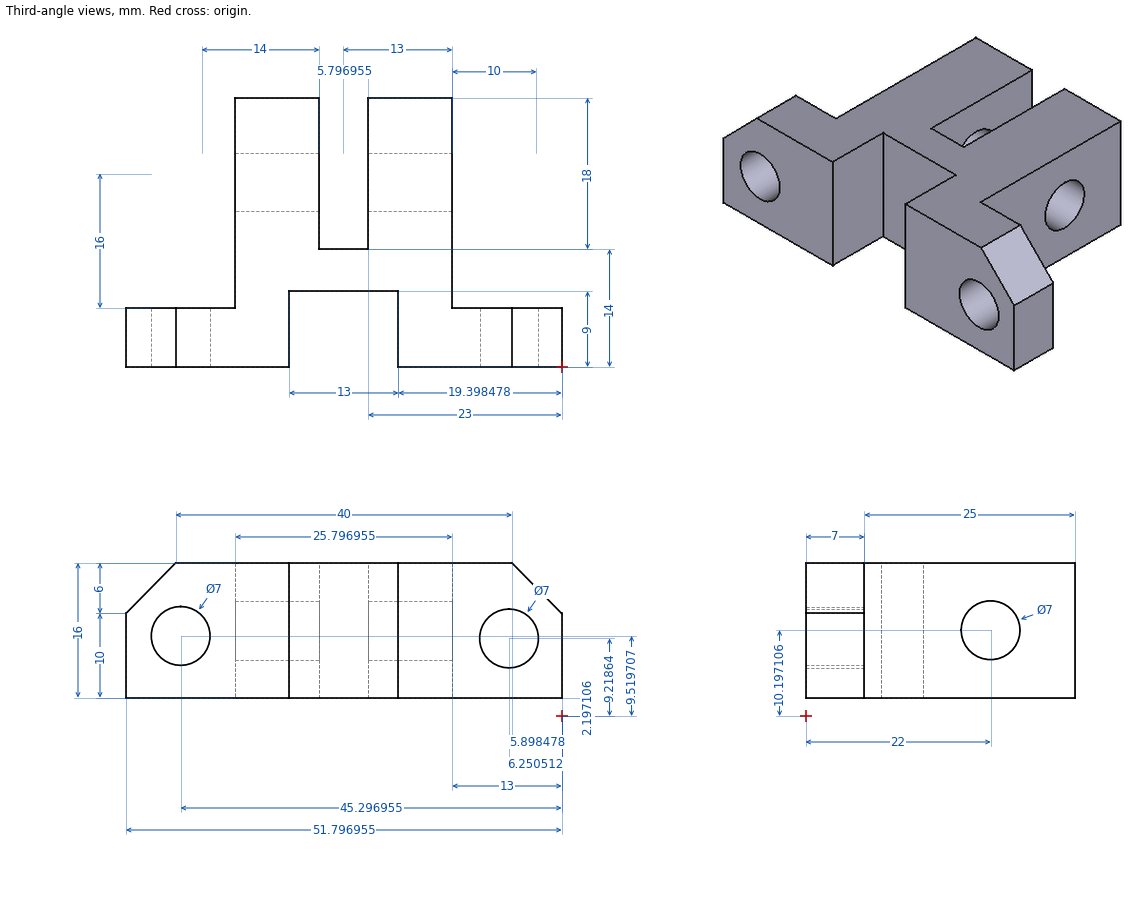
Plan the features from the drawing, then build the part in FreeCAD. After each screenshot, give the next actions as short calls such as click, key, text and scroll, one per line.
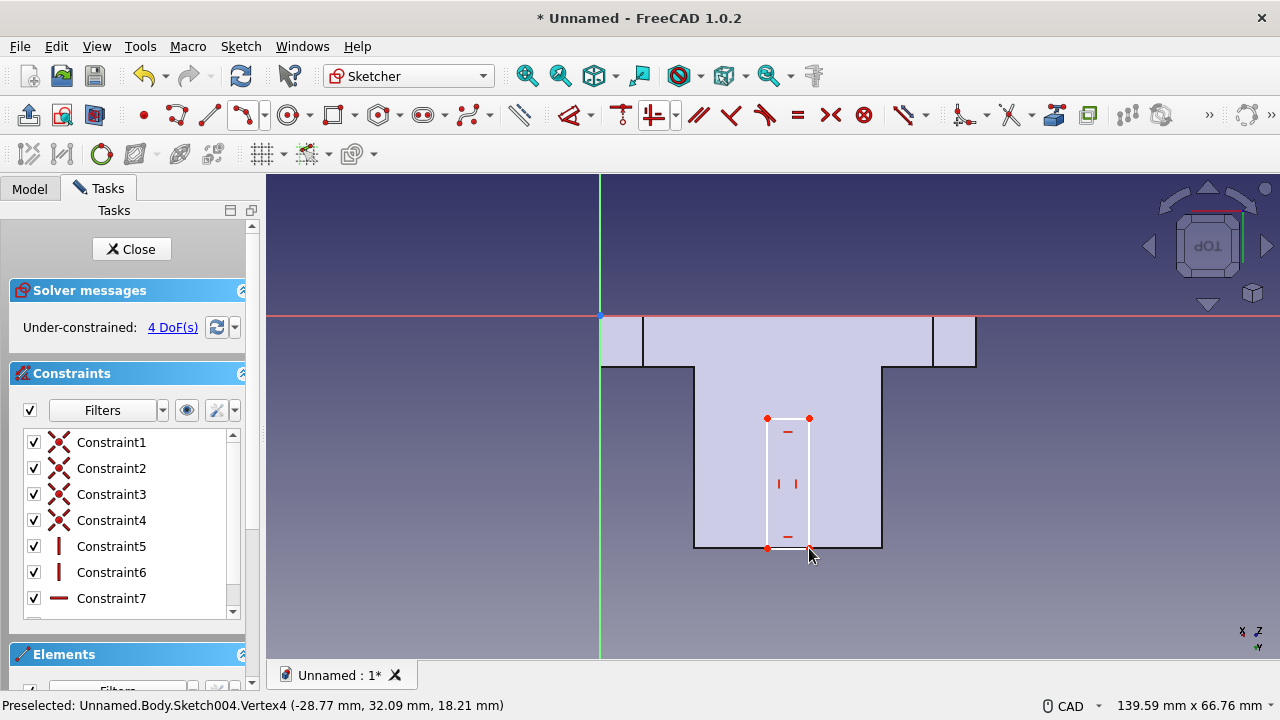
key(d)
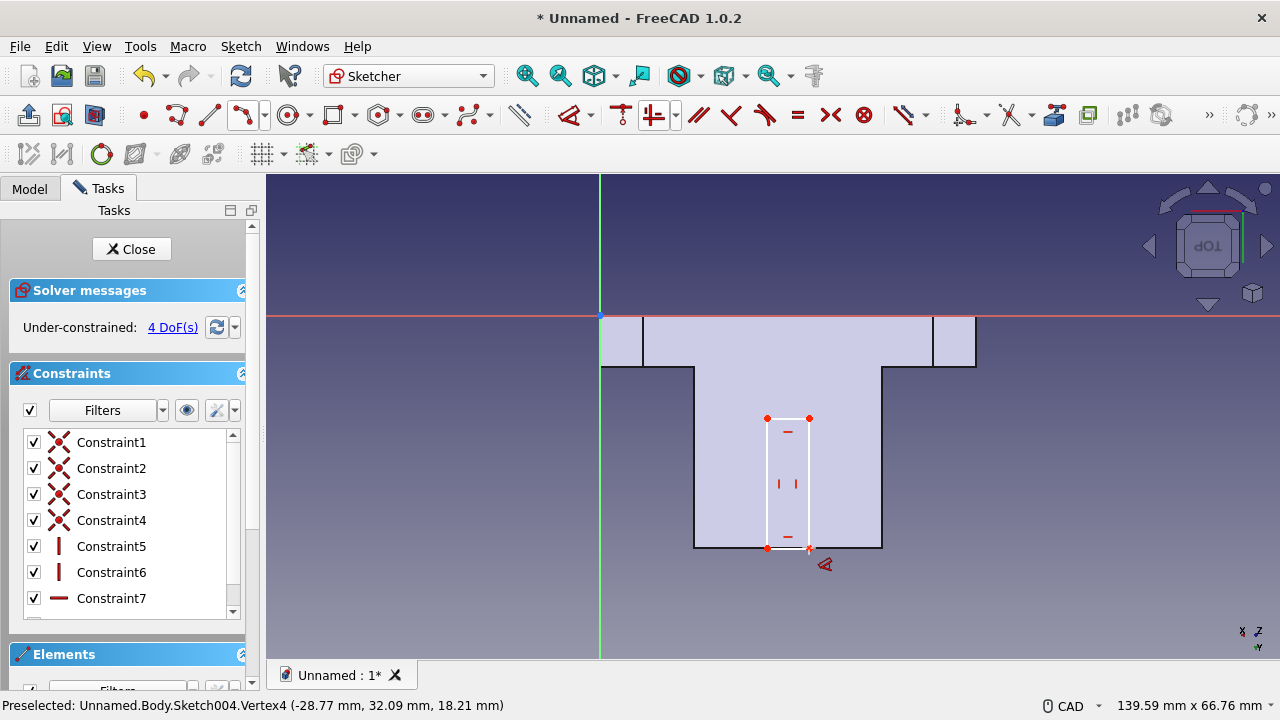
click(767, 458)
click(733, 484)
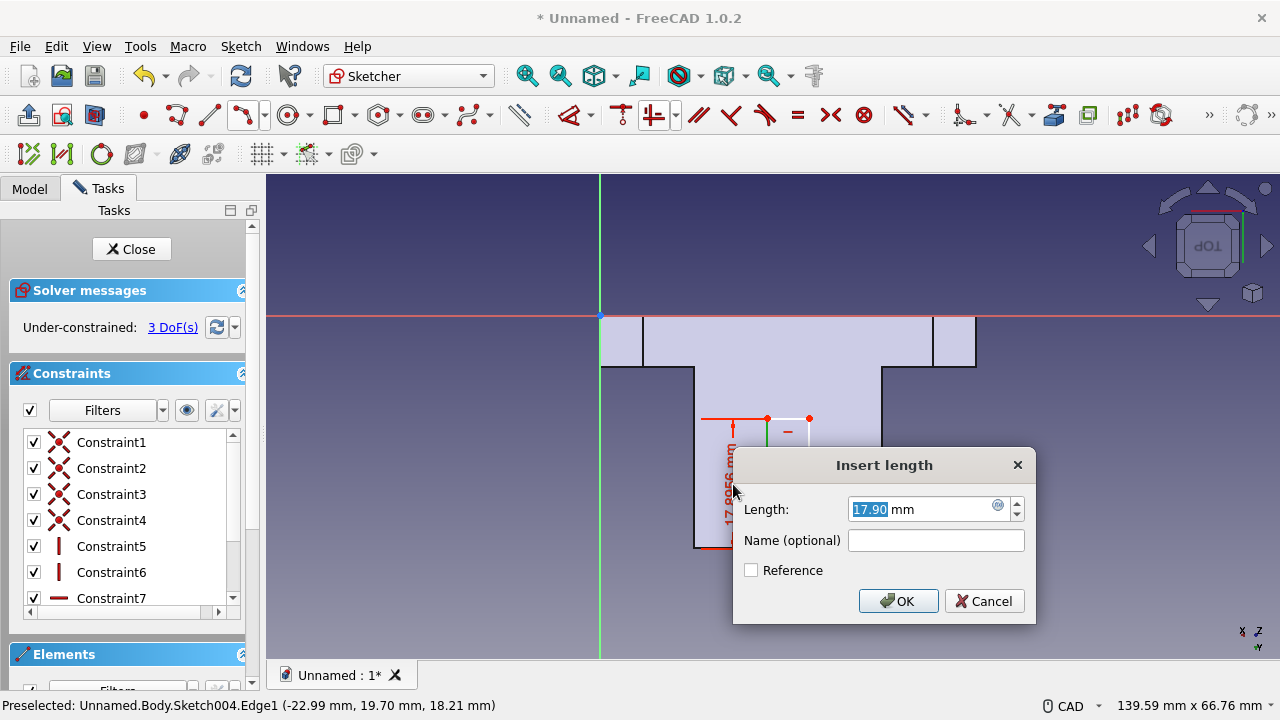
text(18)
key(Return)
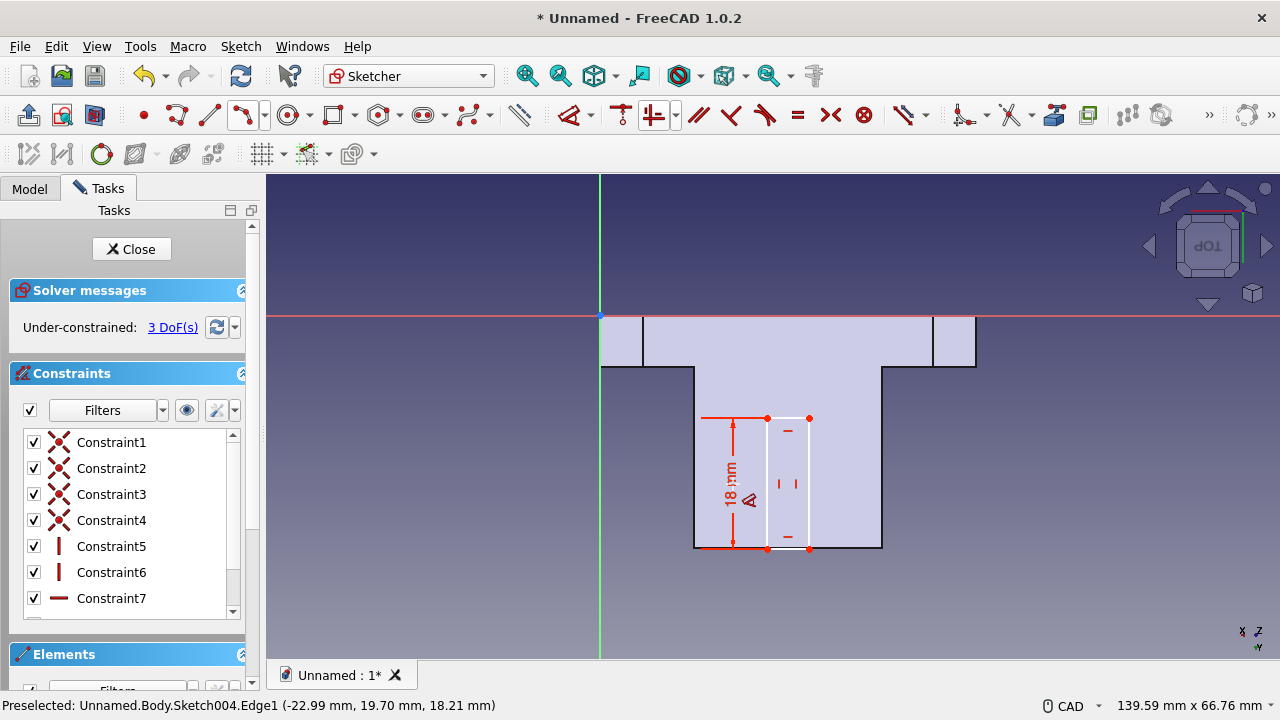
click(767, 418)
click(684, 282)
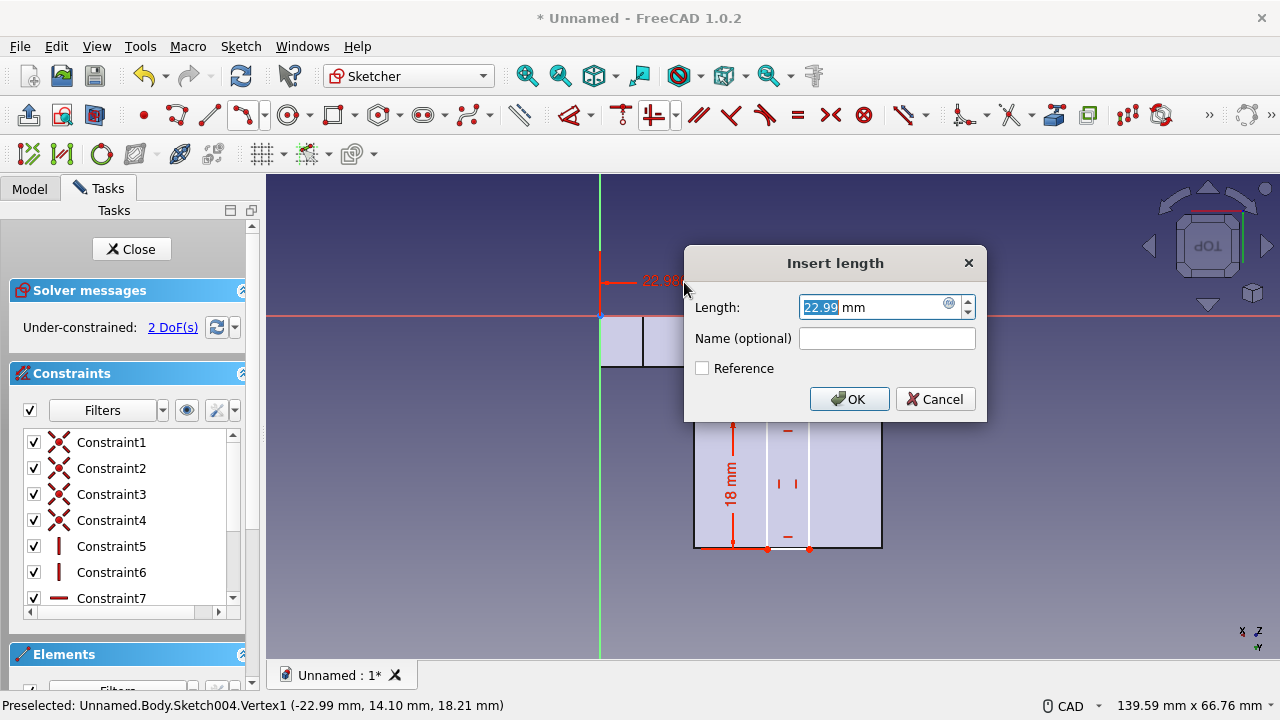
text(23)
key(Return)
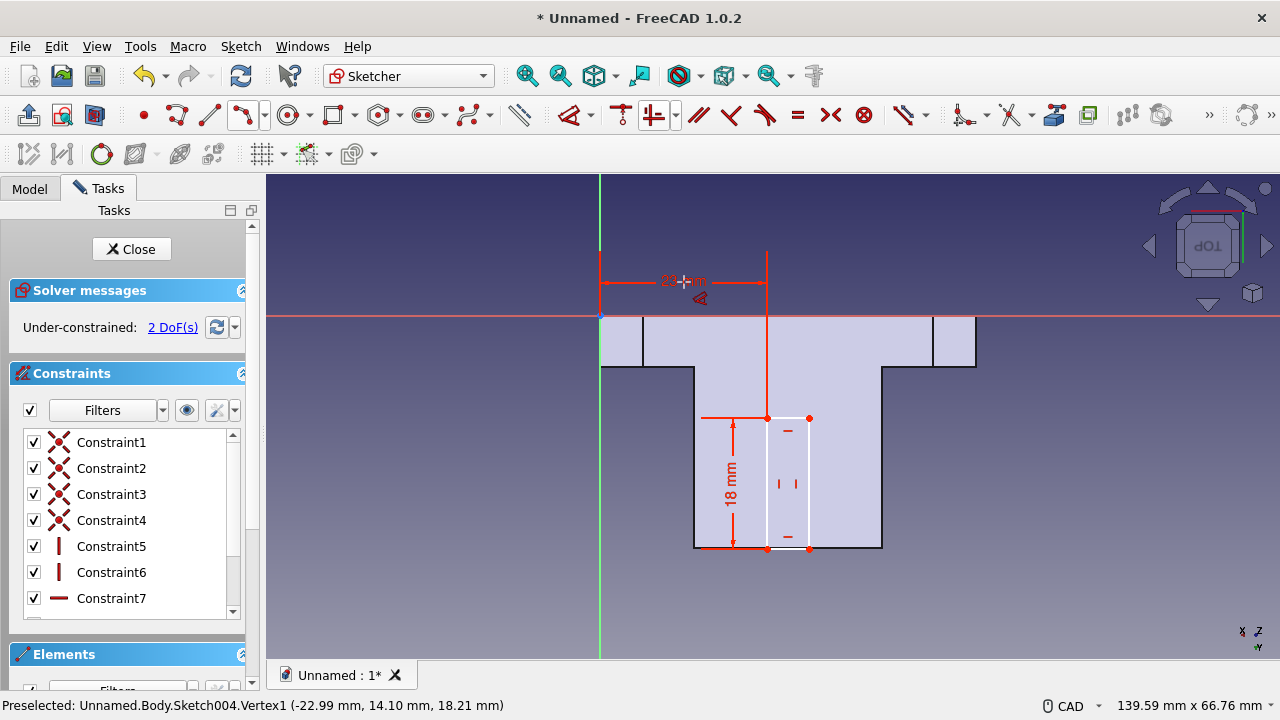
click(767, 418)
click(566, 367)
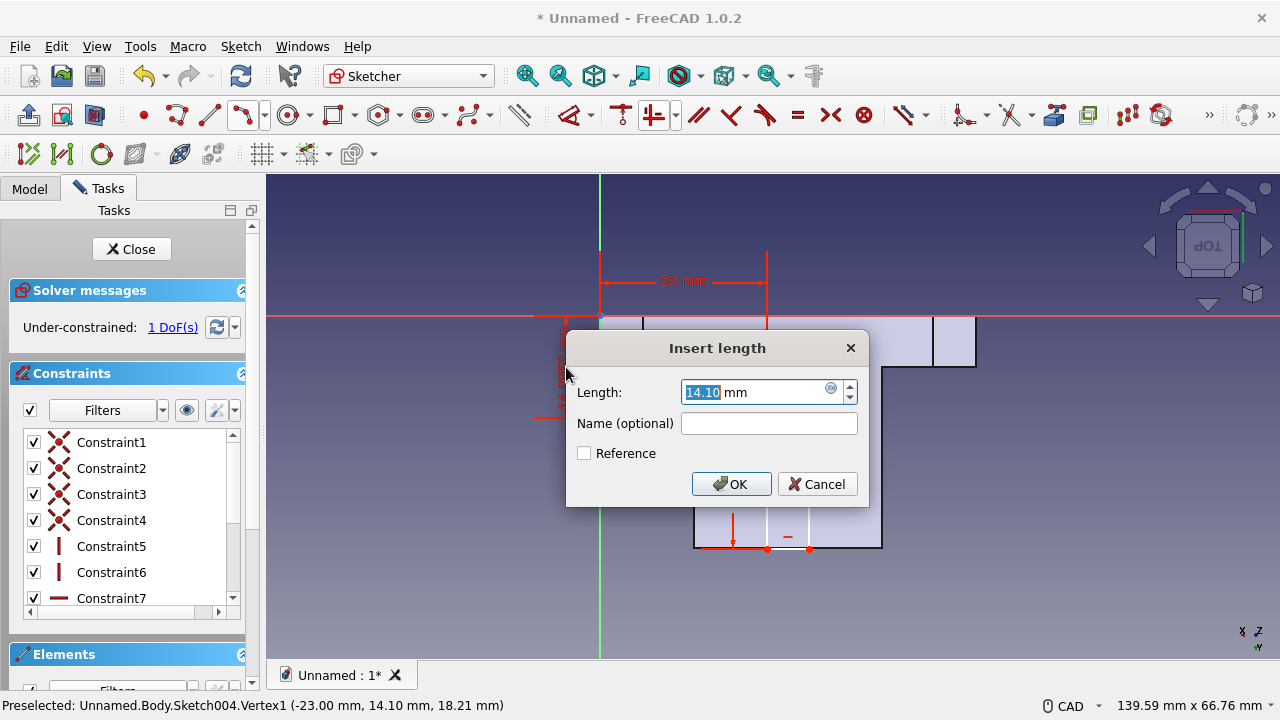
text(14)
key(Return)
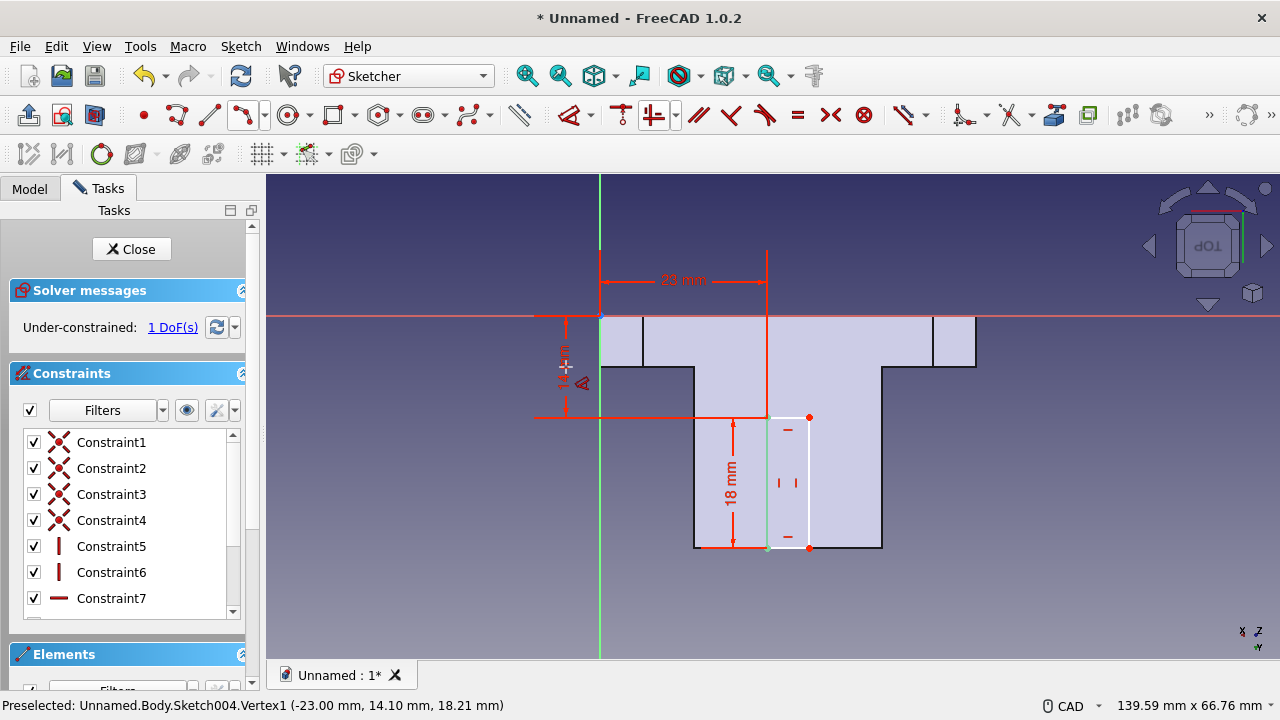
click(780, 548)
click(788, 582)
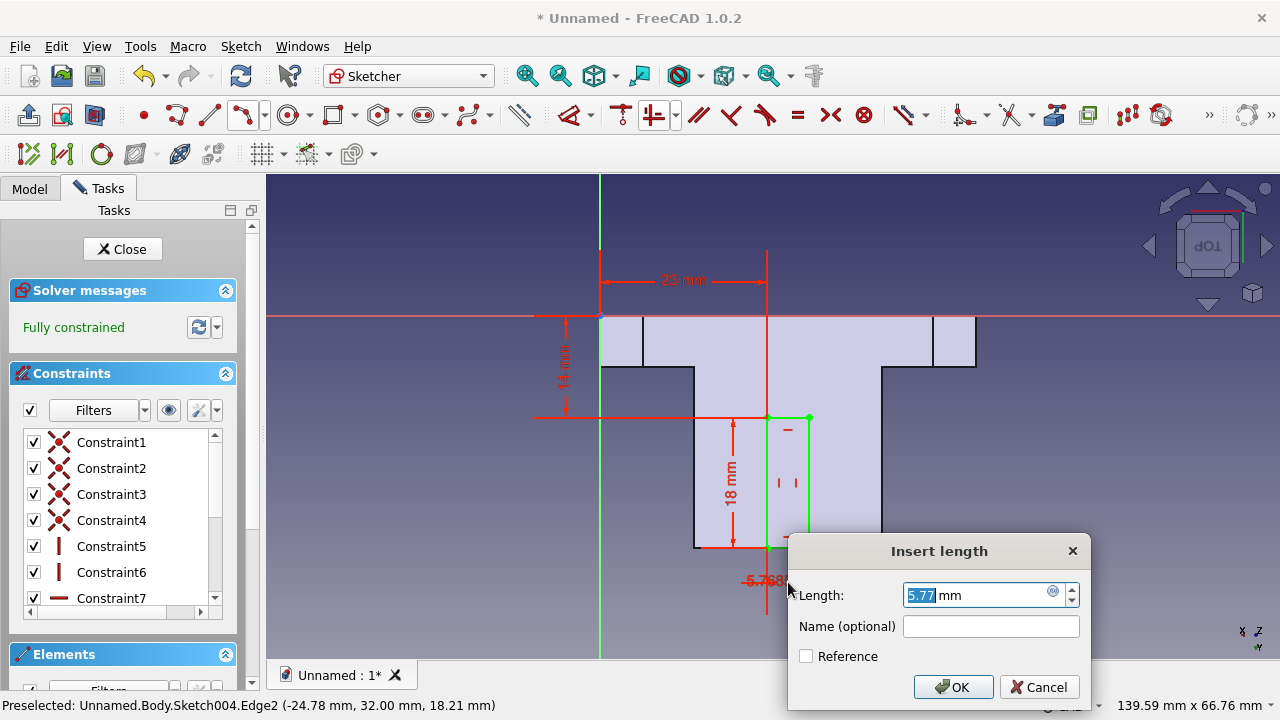
text(5.796955)
key(Return)
key(Escape)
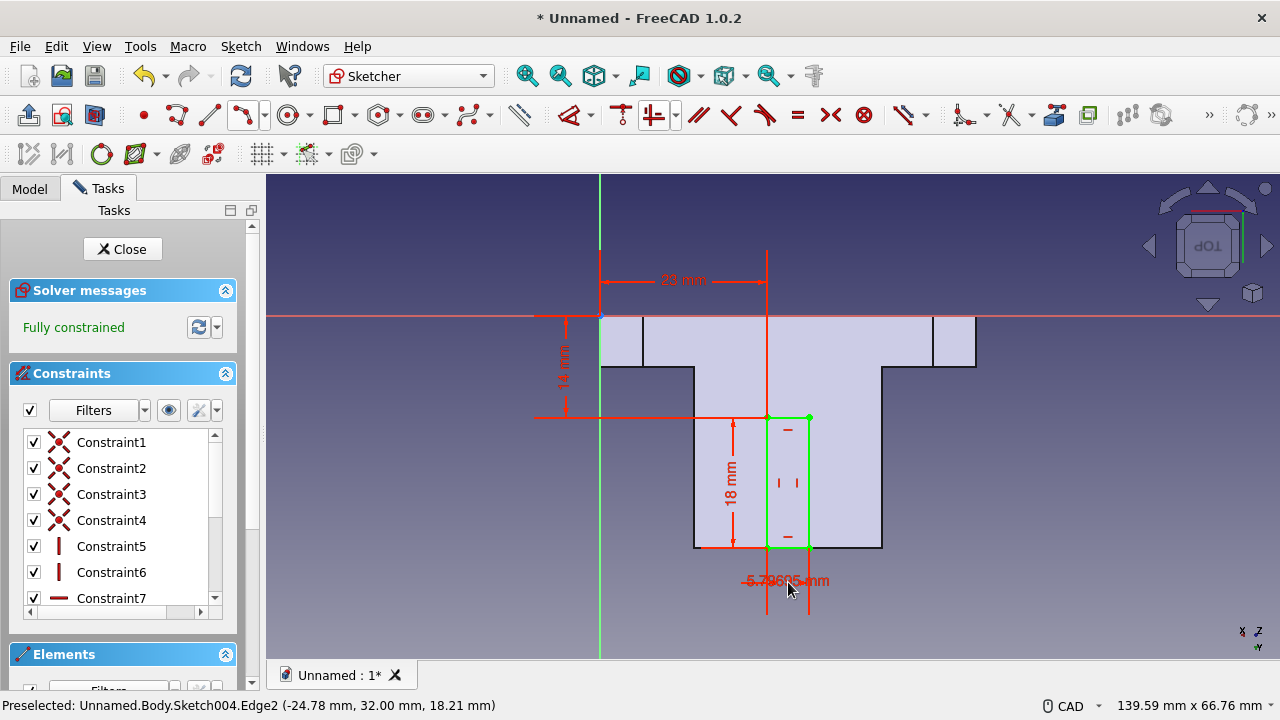
click(123, 249)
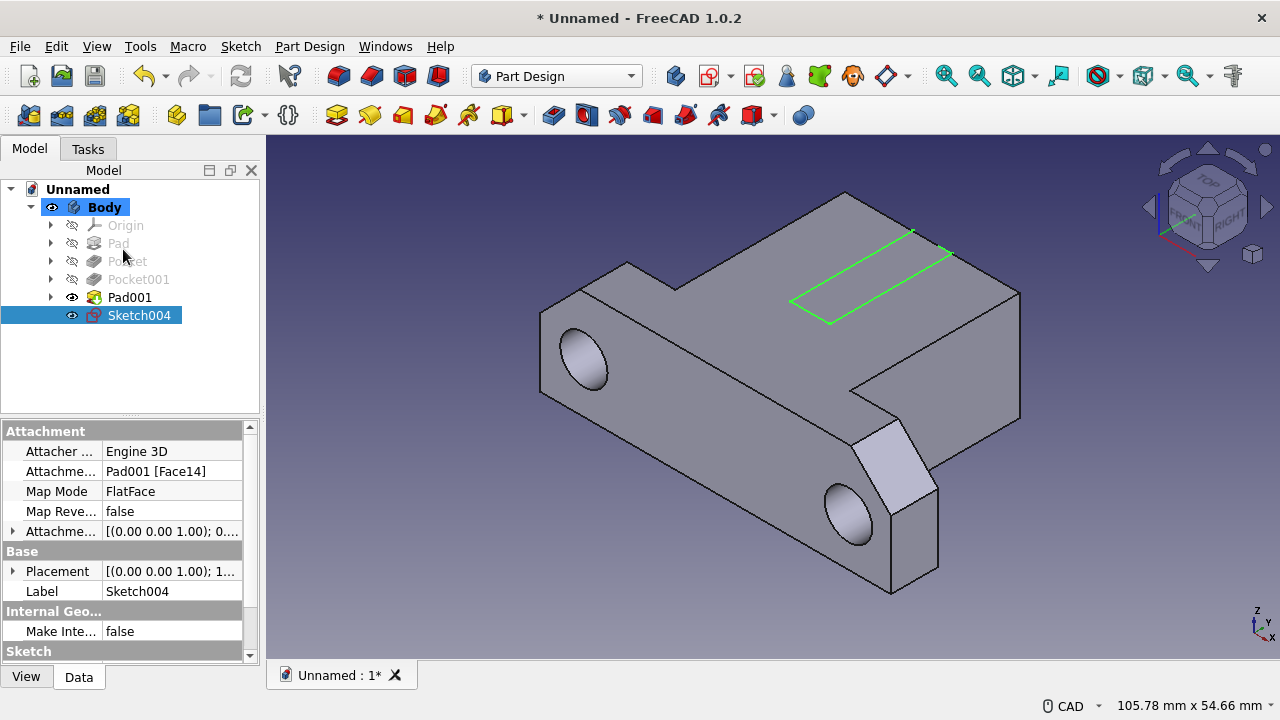
click(554, 116)